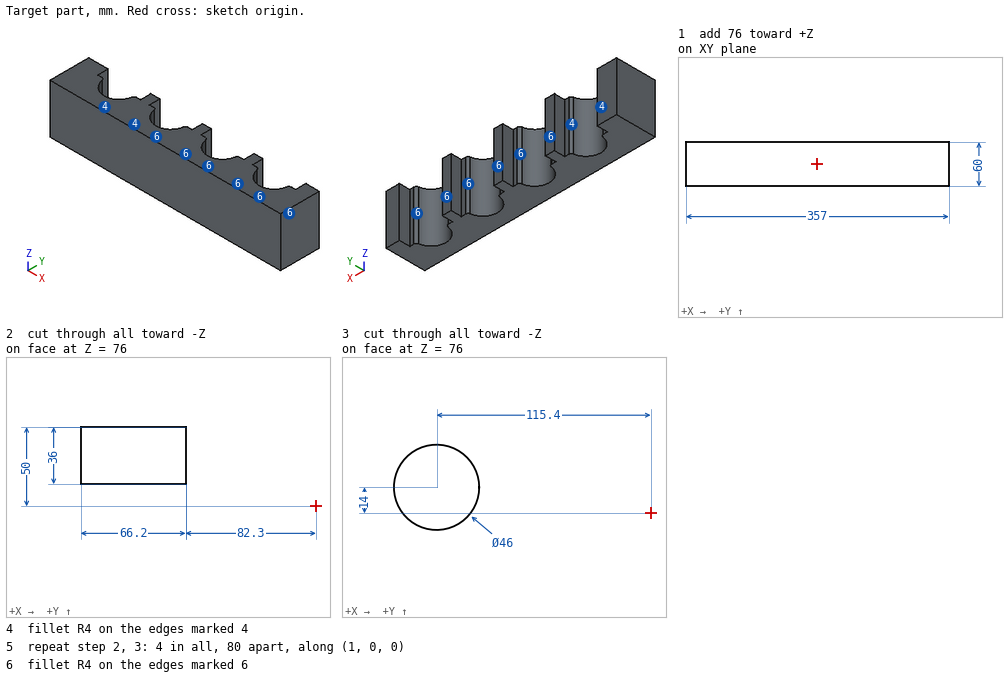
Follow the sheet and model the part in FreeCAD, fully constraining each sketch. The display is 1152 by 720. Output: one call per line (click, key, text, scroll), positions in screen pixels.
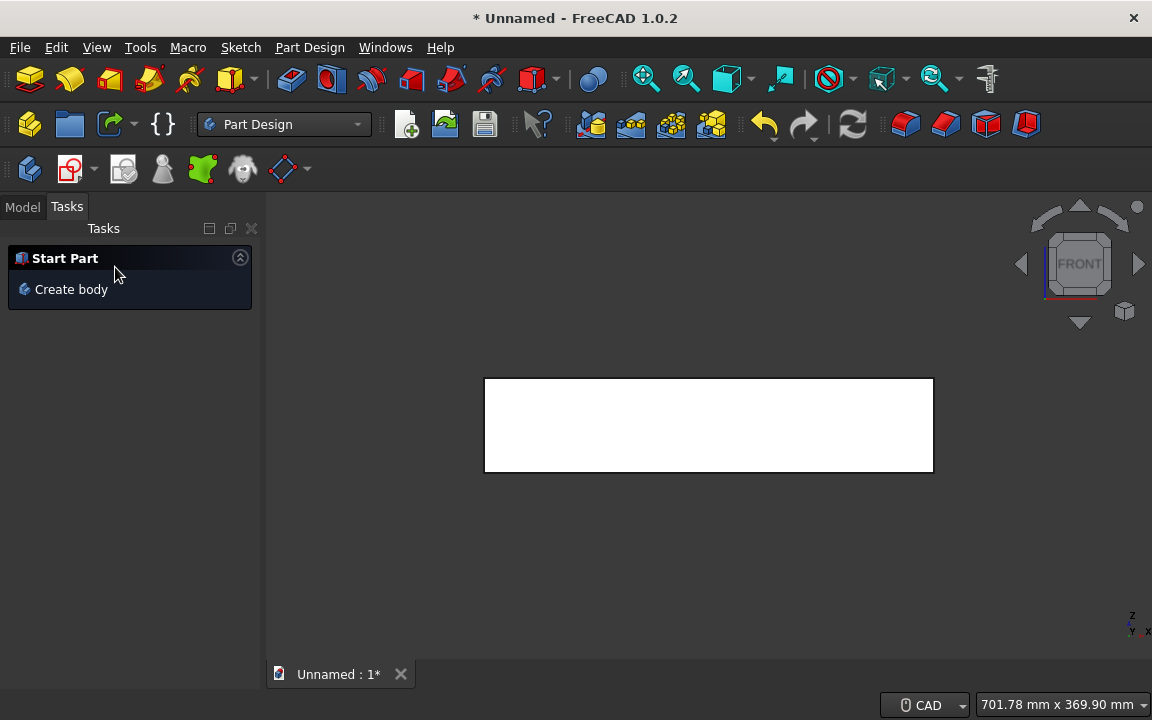
key(3)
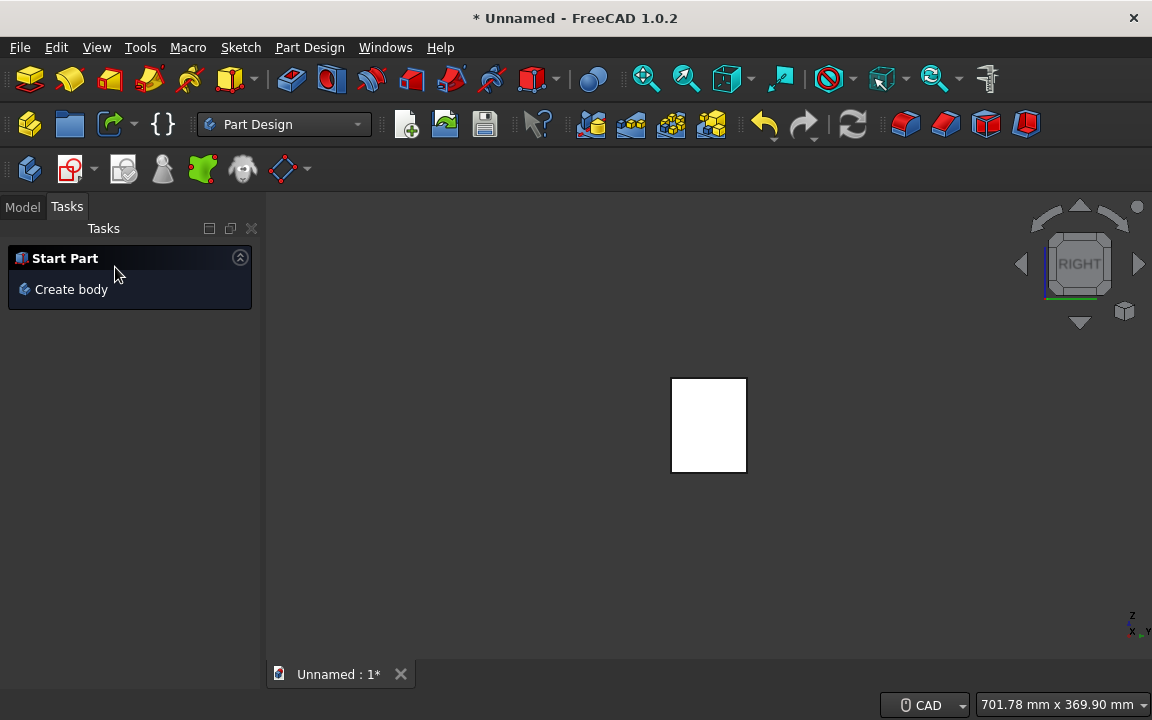
key(v)
key(f)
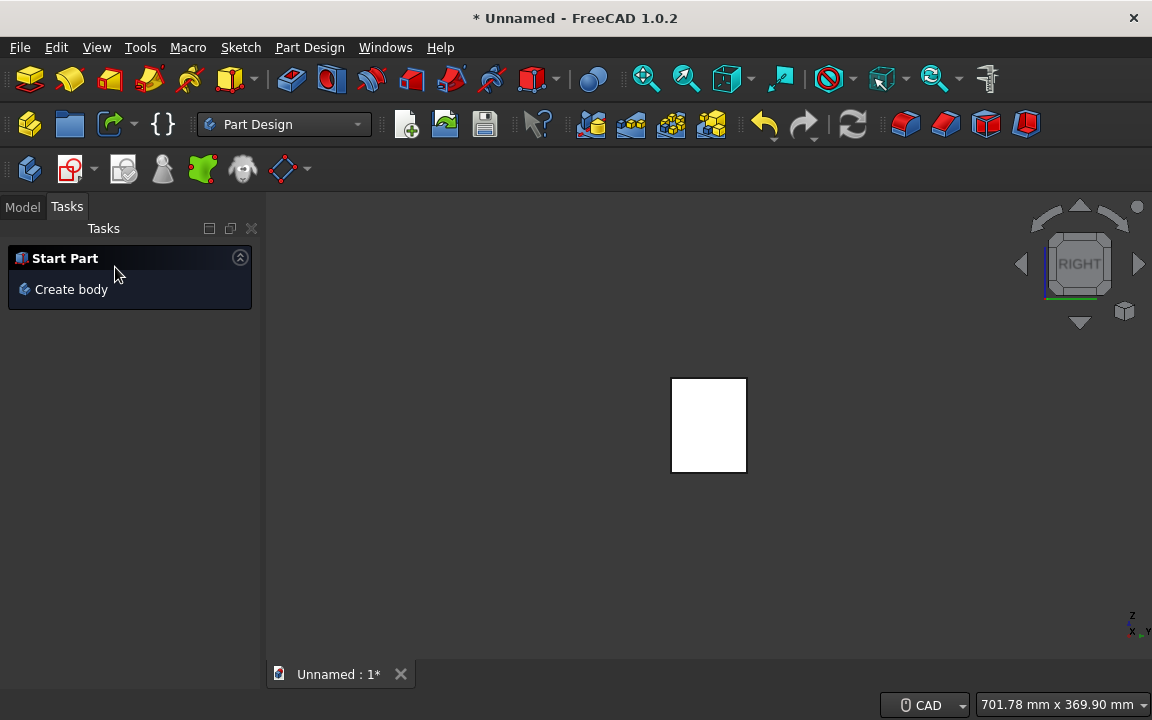
key(5)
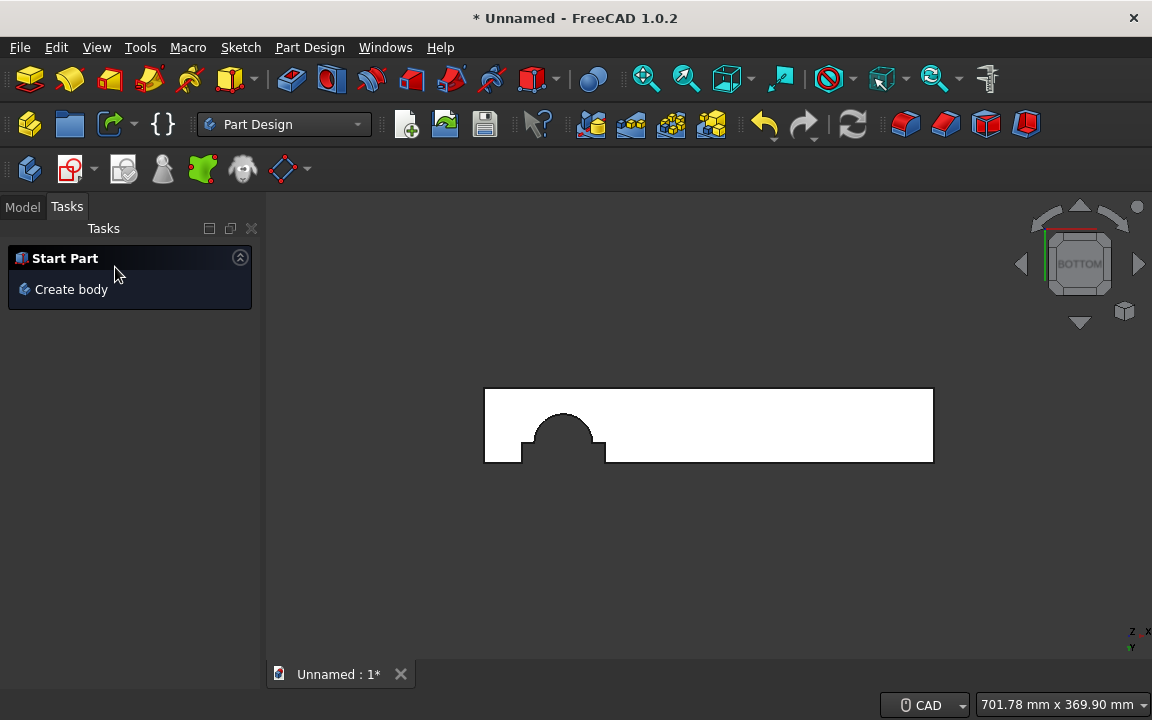
key(4)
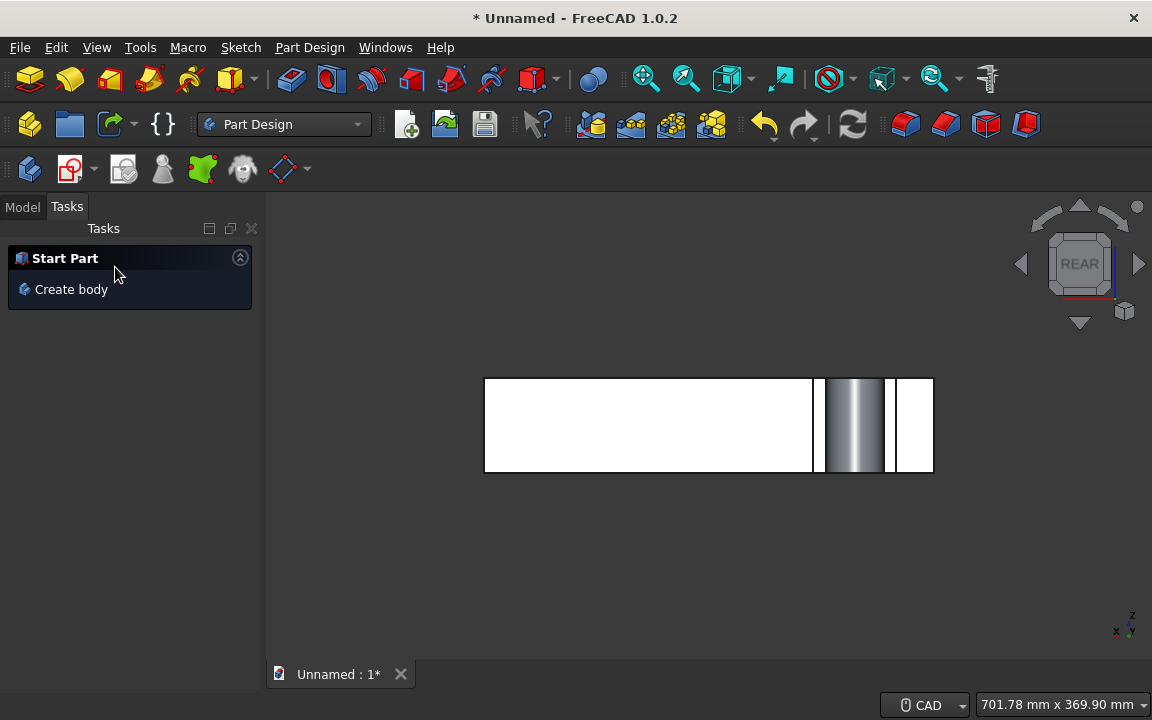
click(884, 424)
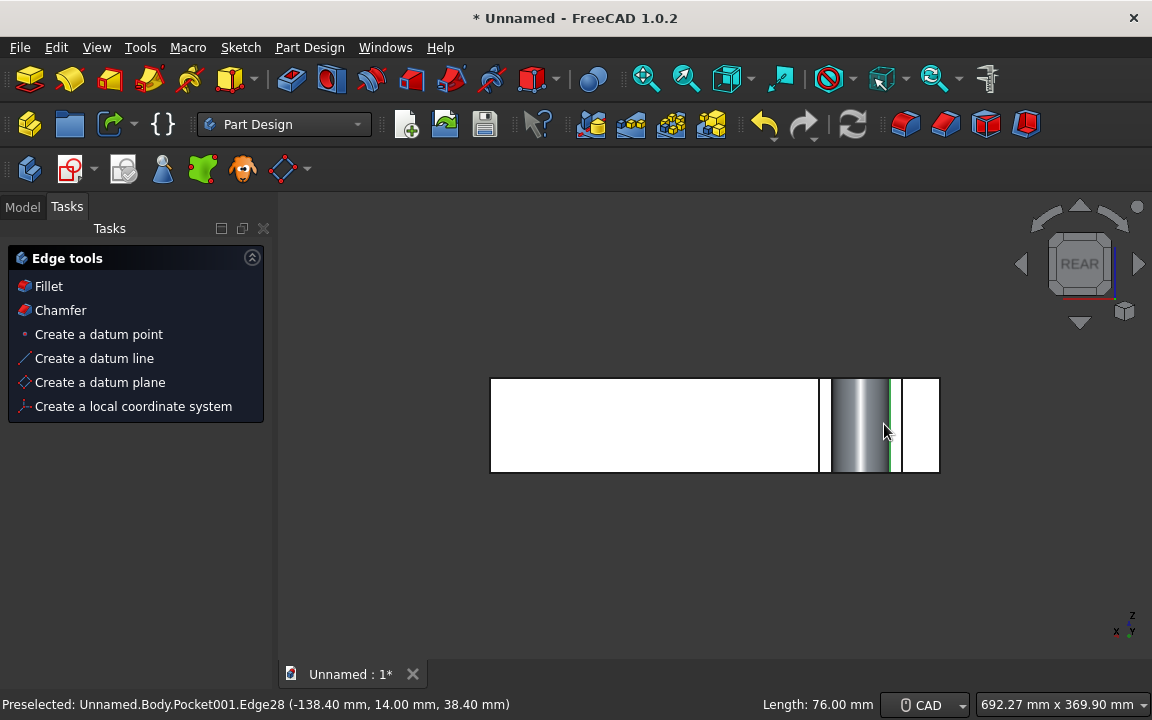
click(832, 424, ctrl)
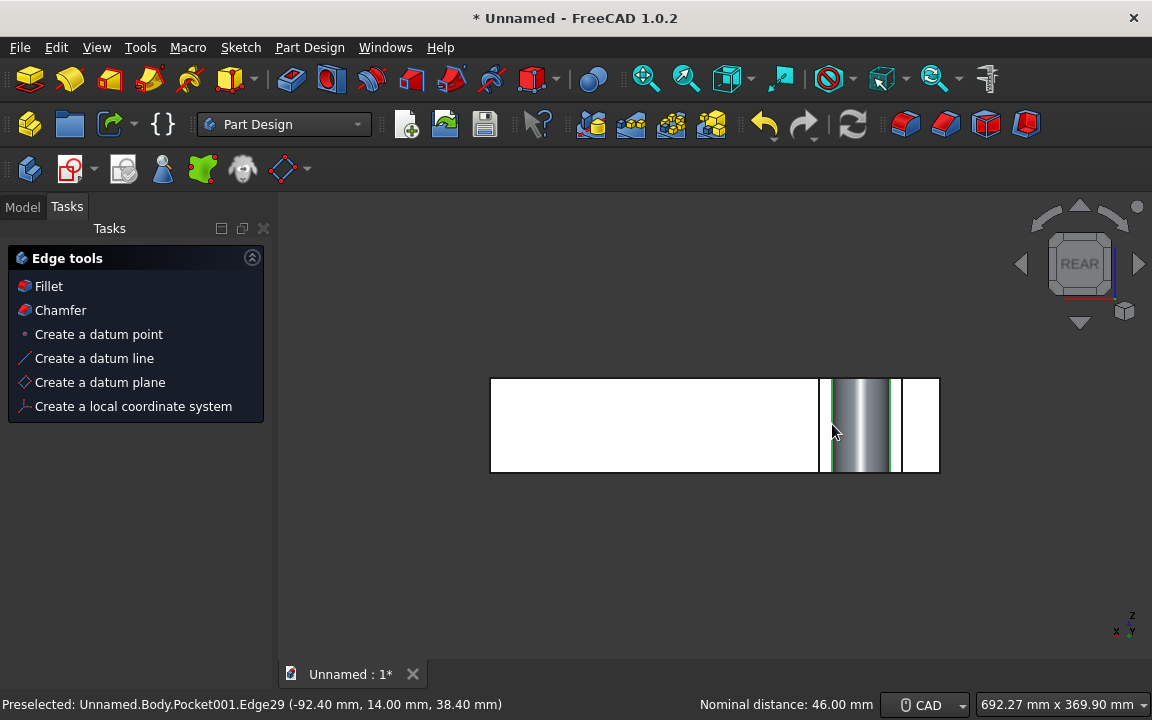
click(906, 124)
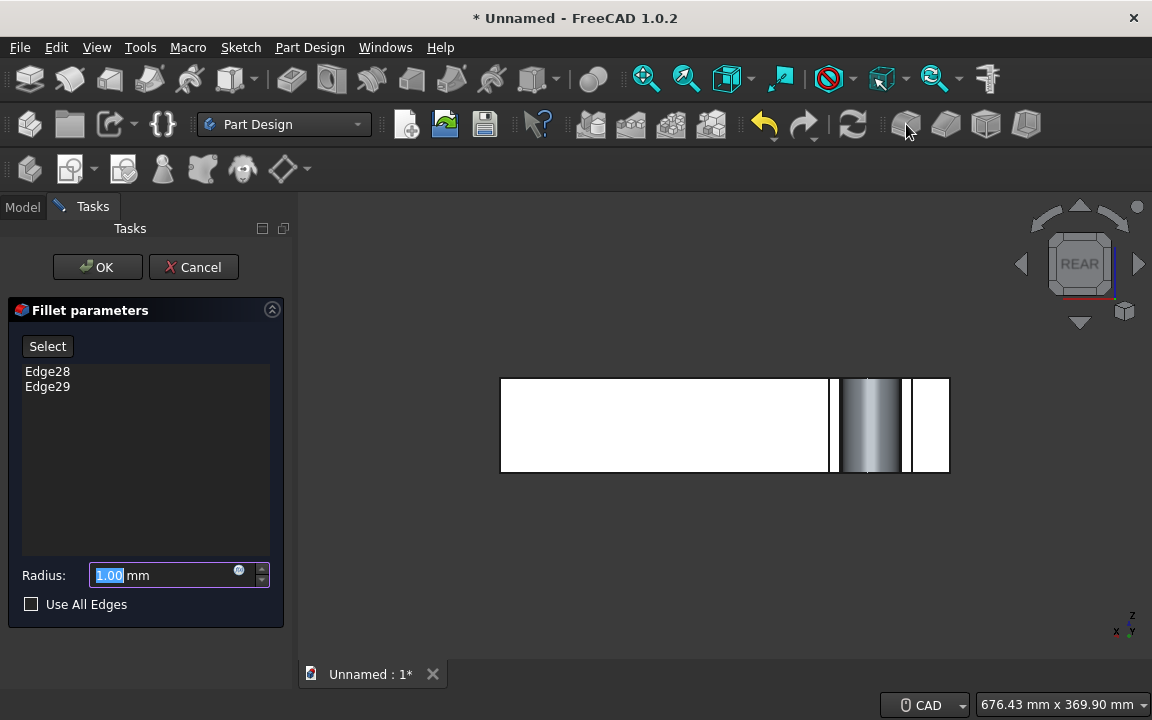
text(4)
key(Tab)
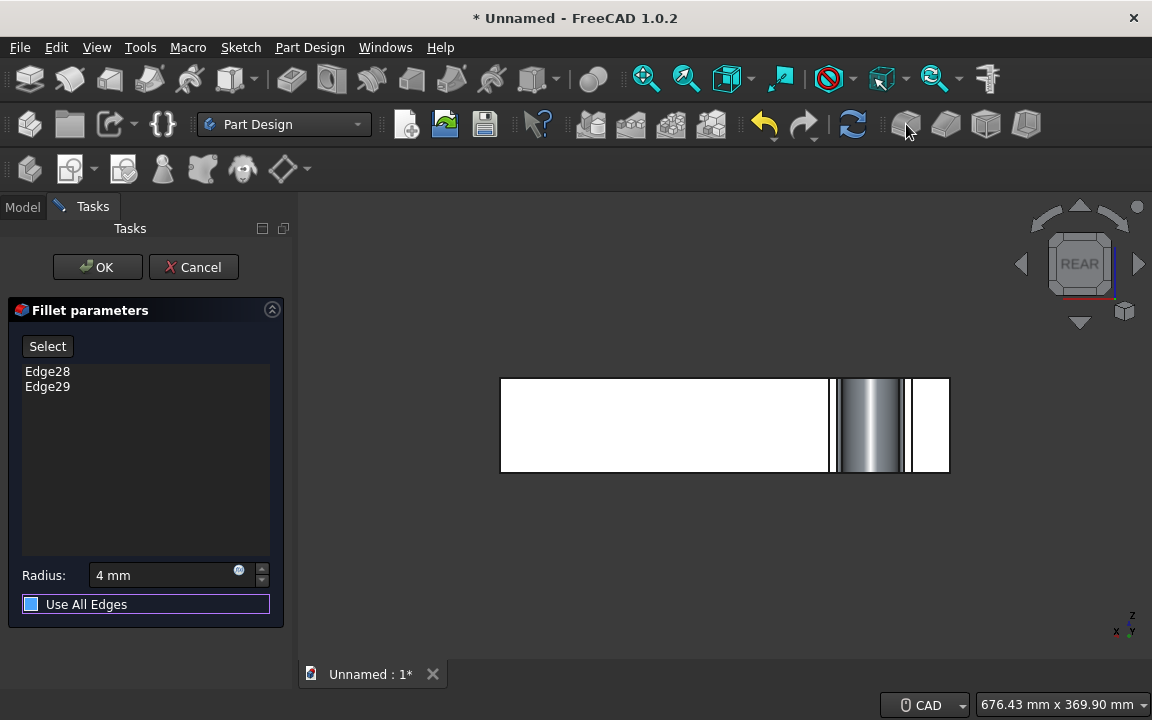
click(98, 267)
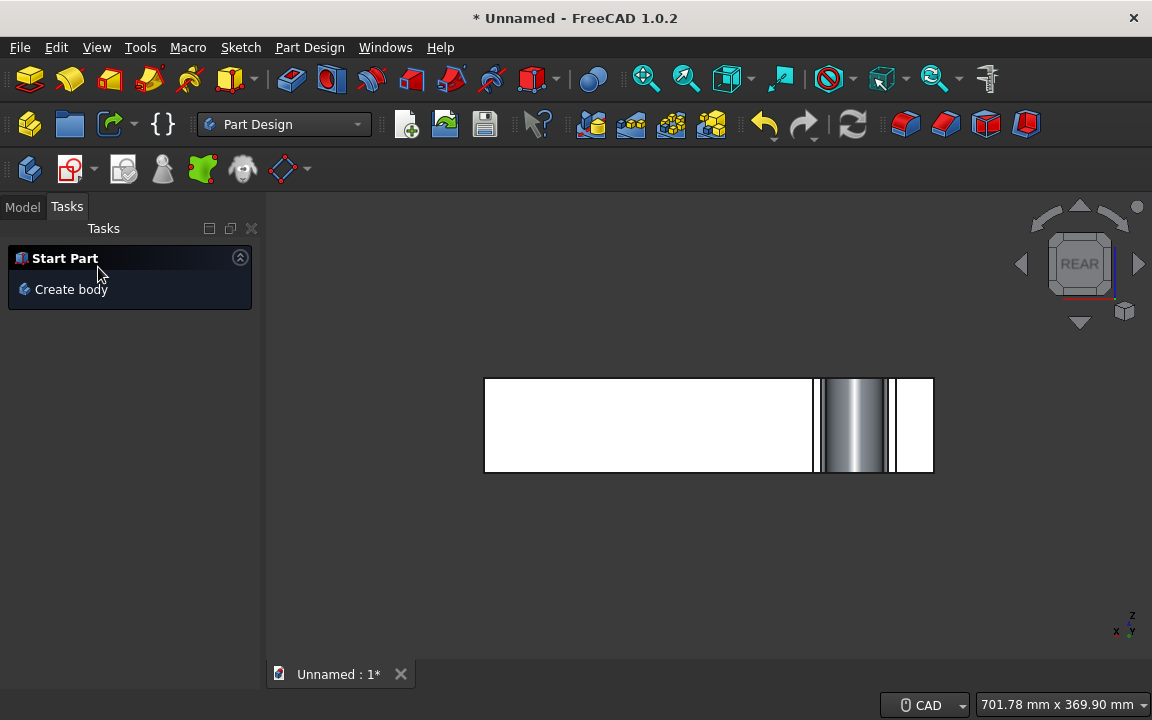
click(23, 206)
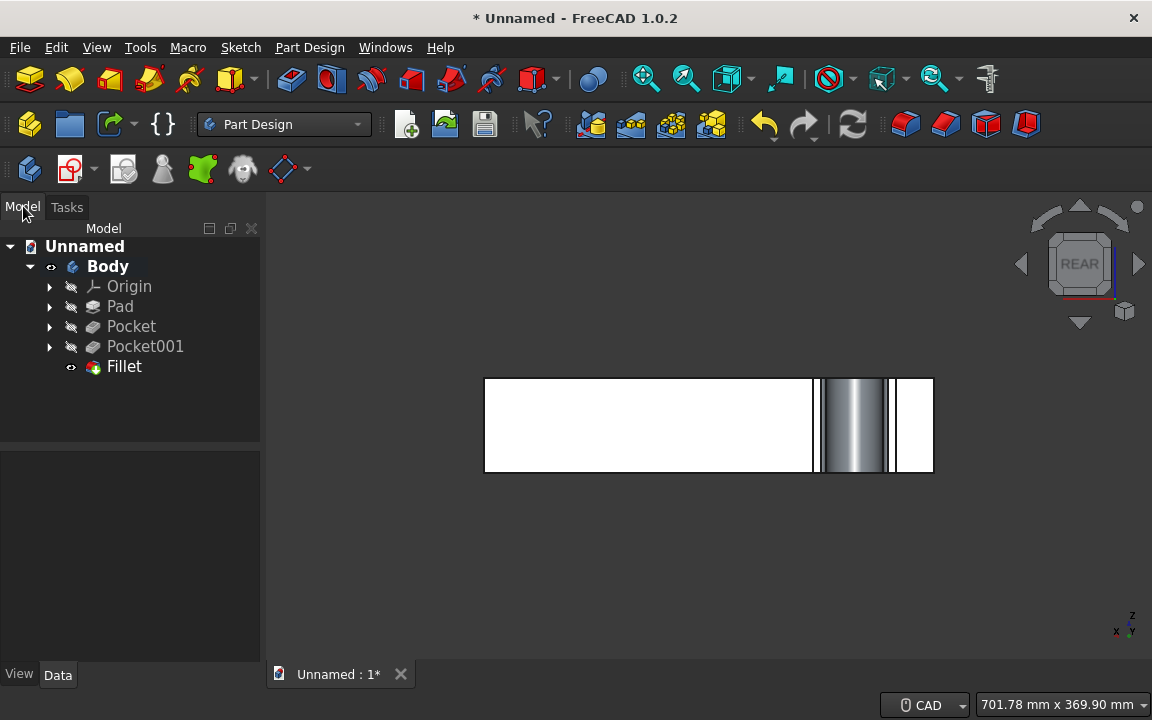
click(116, 327)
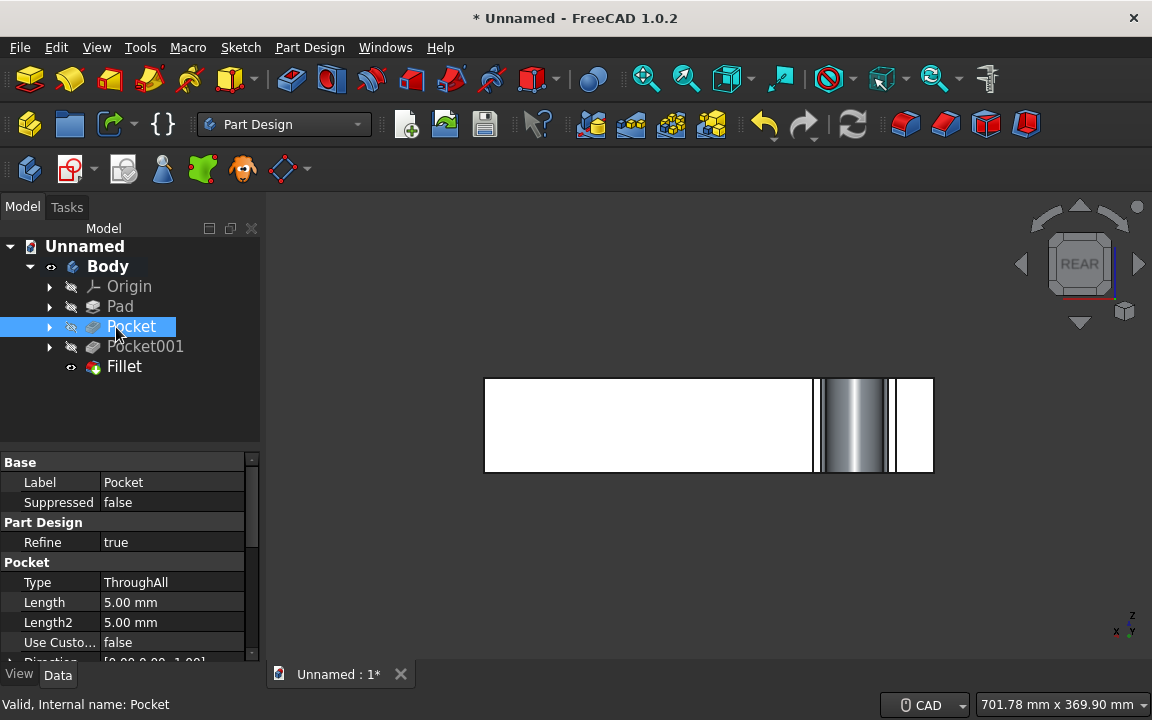
click(116, 347, ctrl)